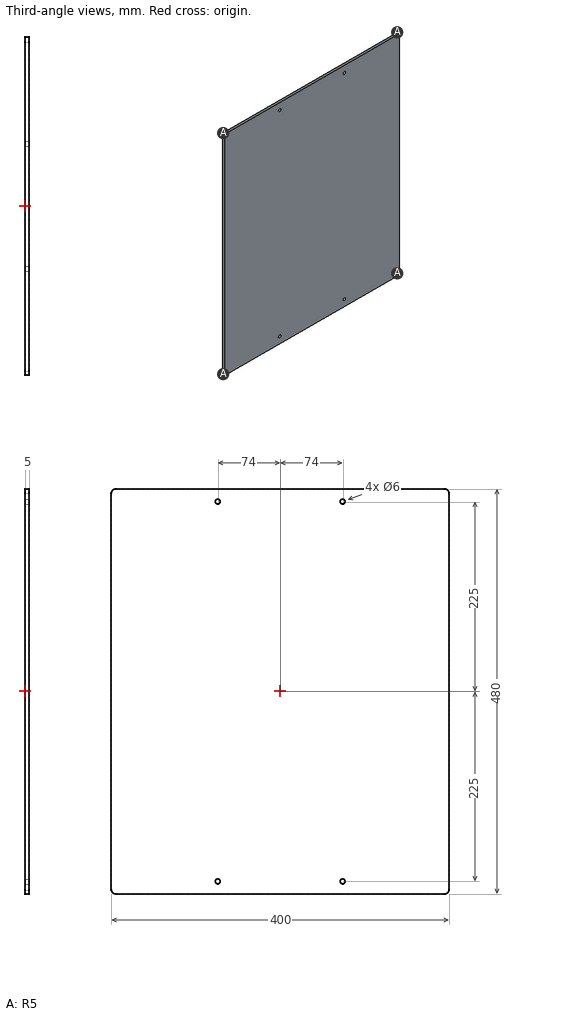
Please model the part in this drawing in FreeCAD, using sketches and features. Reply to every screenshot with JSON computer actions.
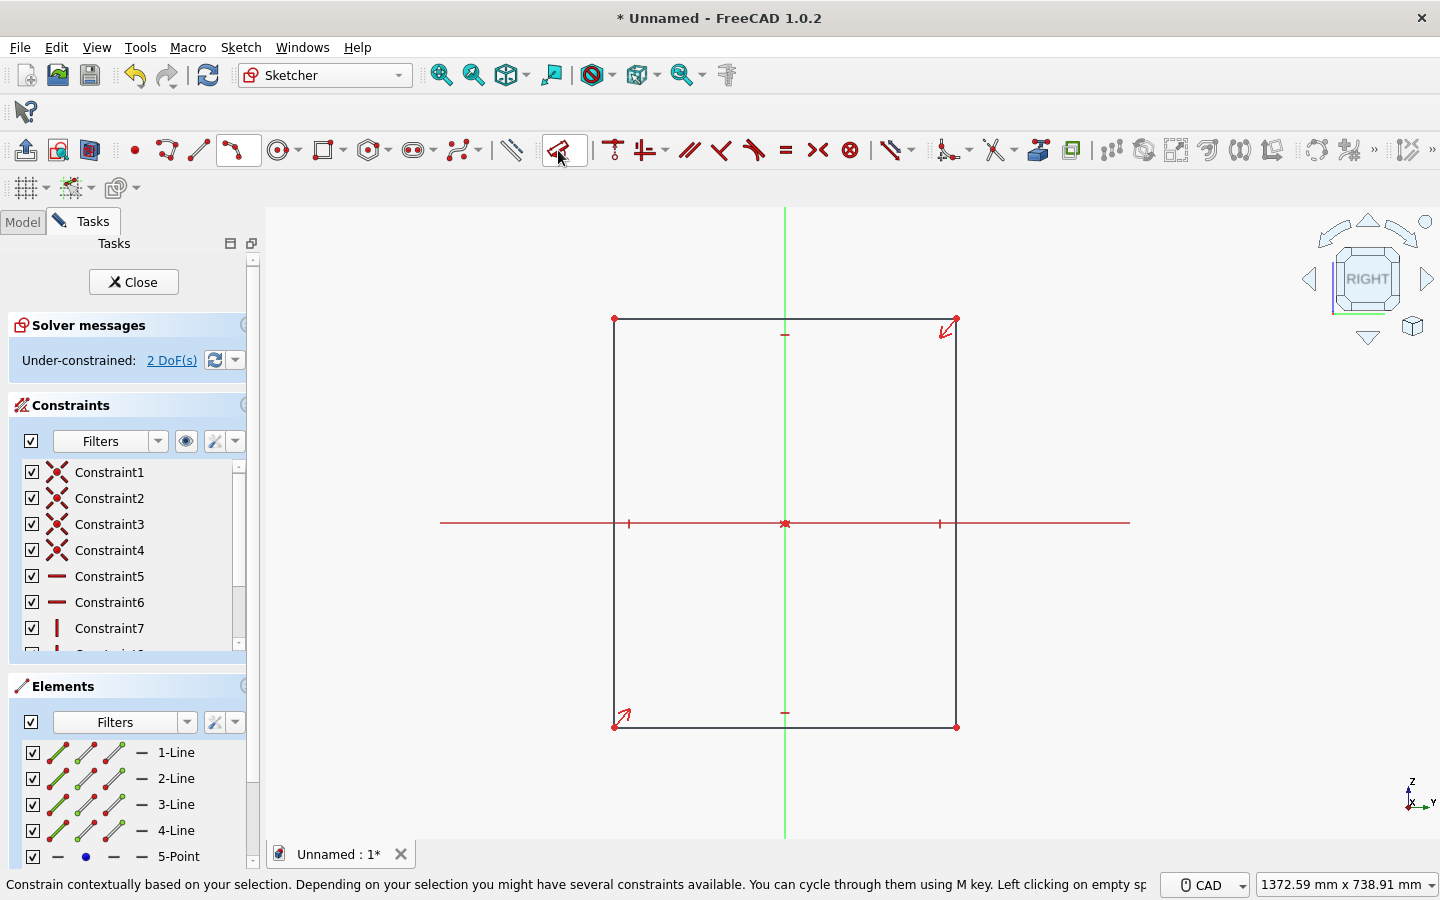
{"action": "left_click", "coordinate": [717, 728]}
{"action": "left_click", "coordinate": [706, 762]}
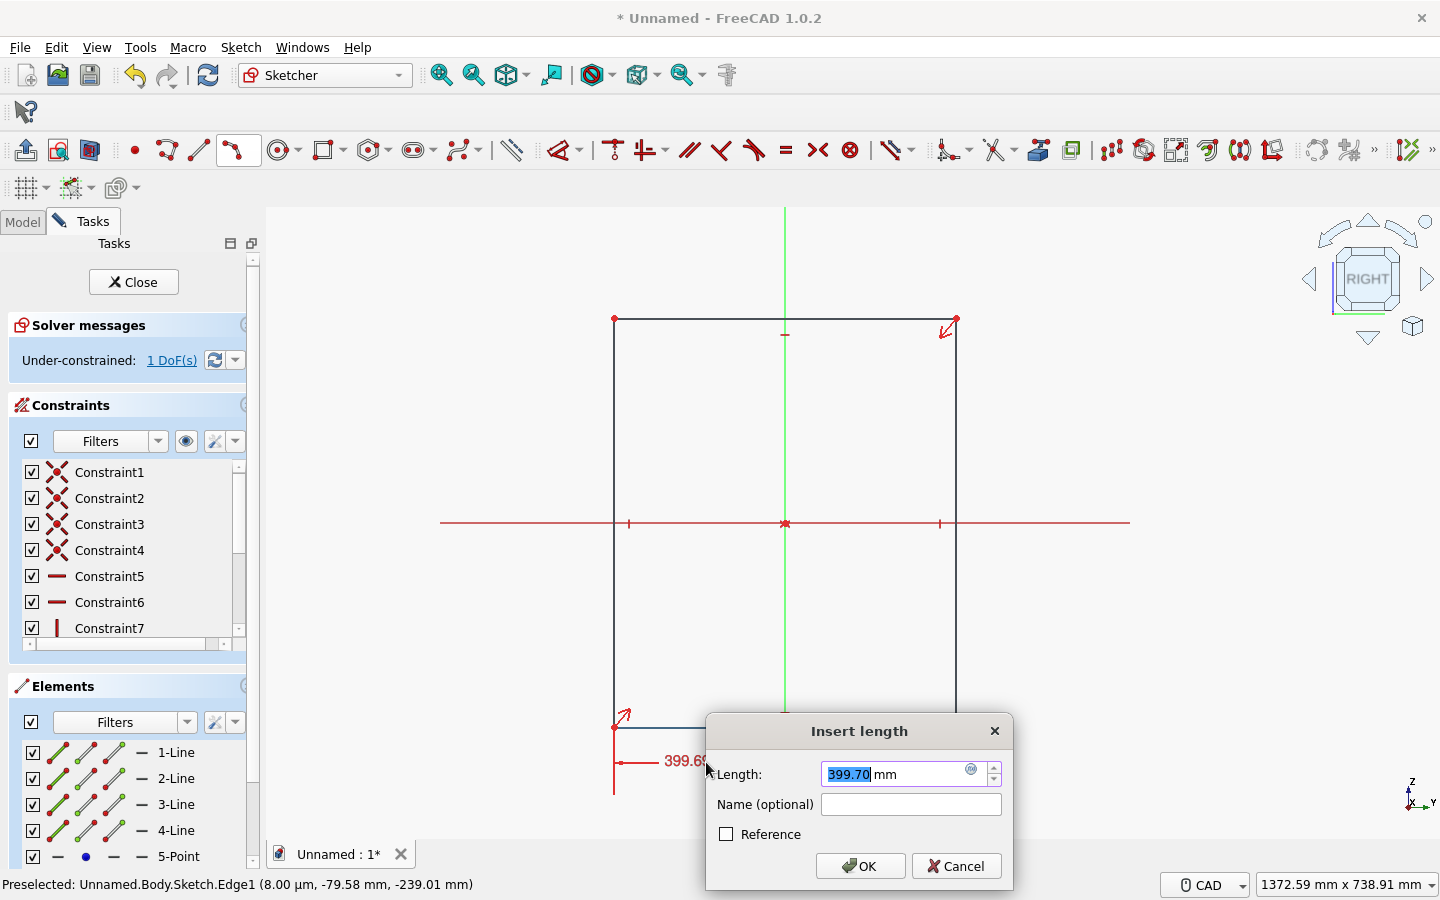
{"action": "type", "text": "400"}
{"action": "key", "text": "Return"}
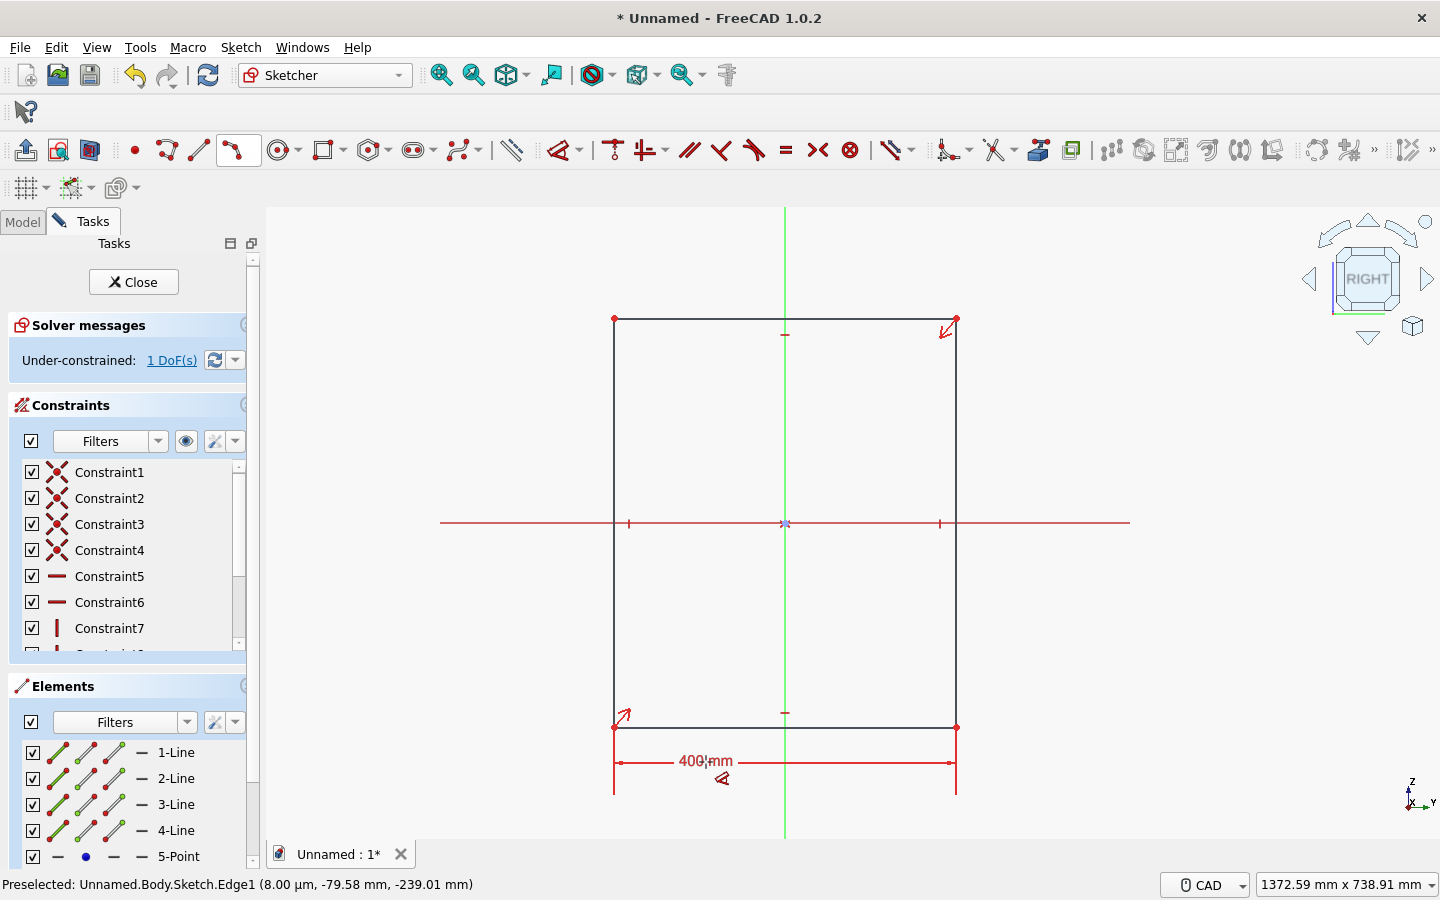
{"action": "left_click", "coordinate": [956, 605]}
{"action": "left_click", "coordinate": [990, 429]}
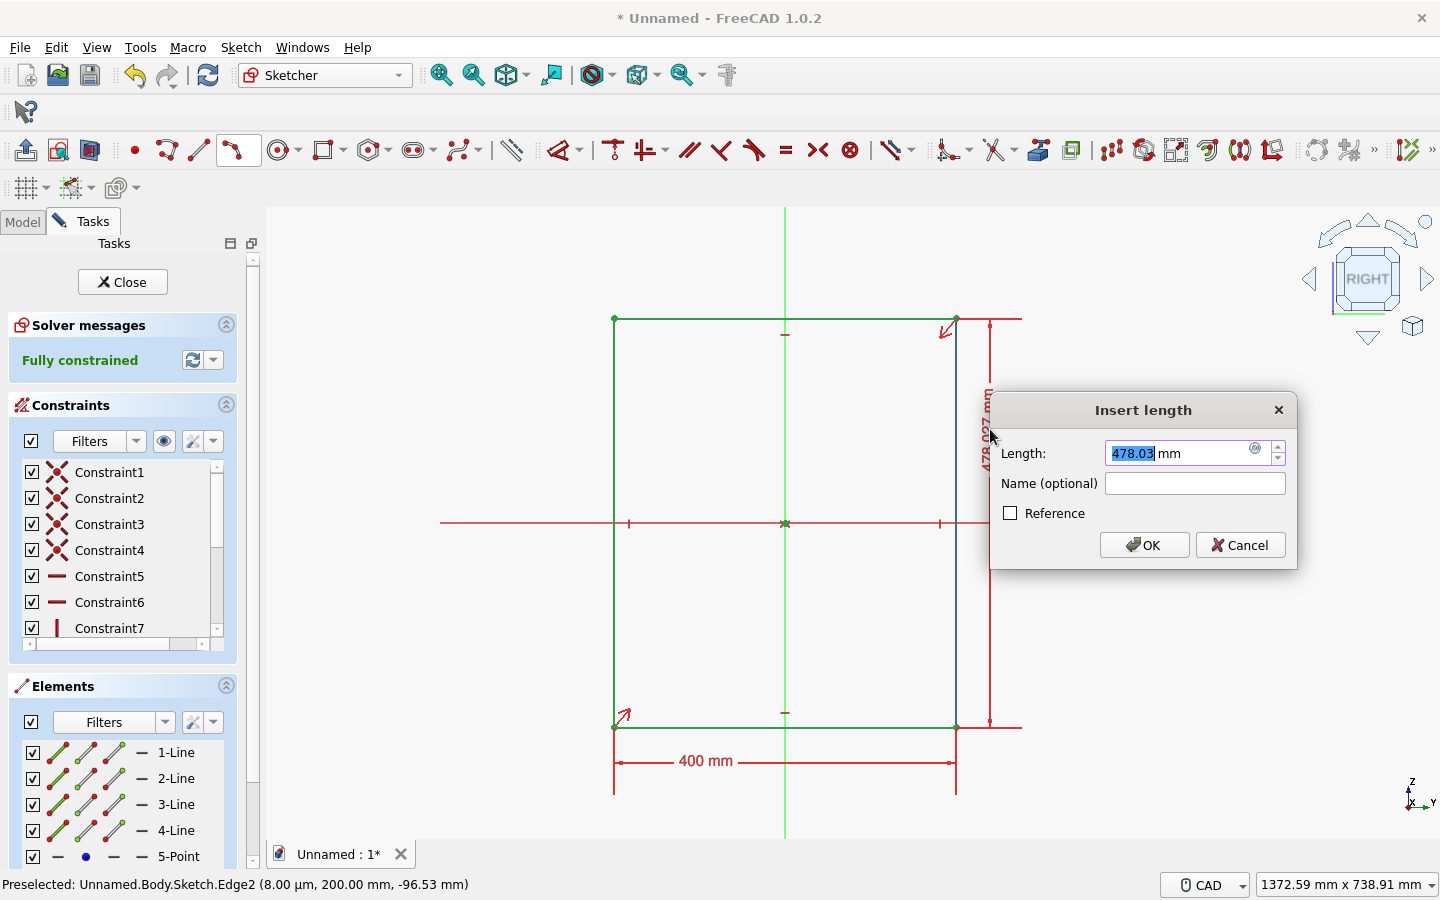
{"action": "type", "text": "480"}
{"action": "key", "text": "Return"}
{"action": "key", "text": "Escape"}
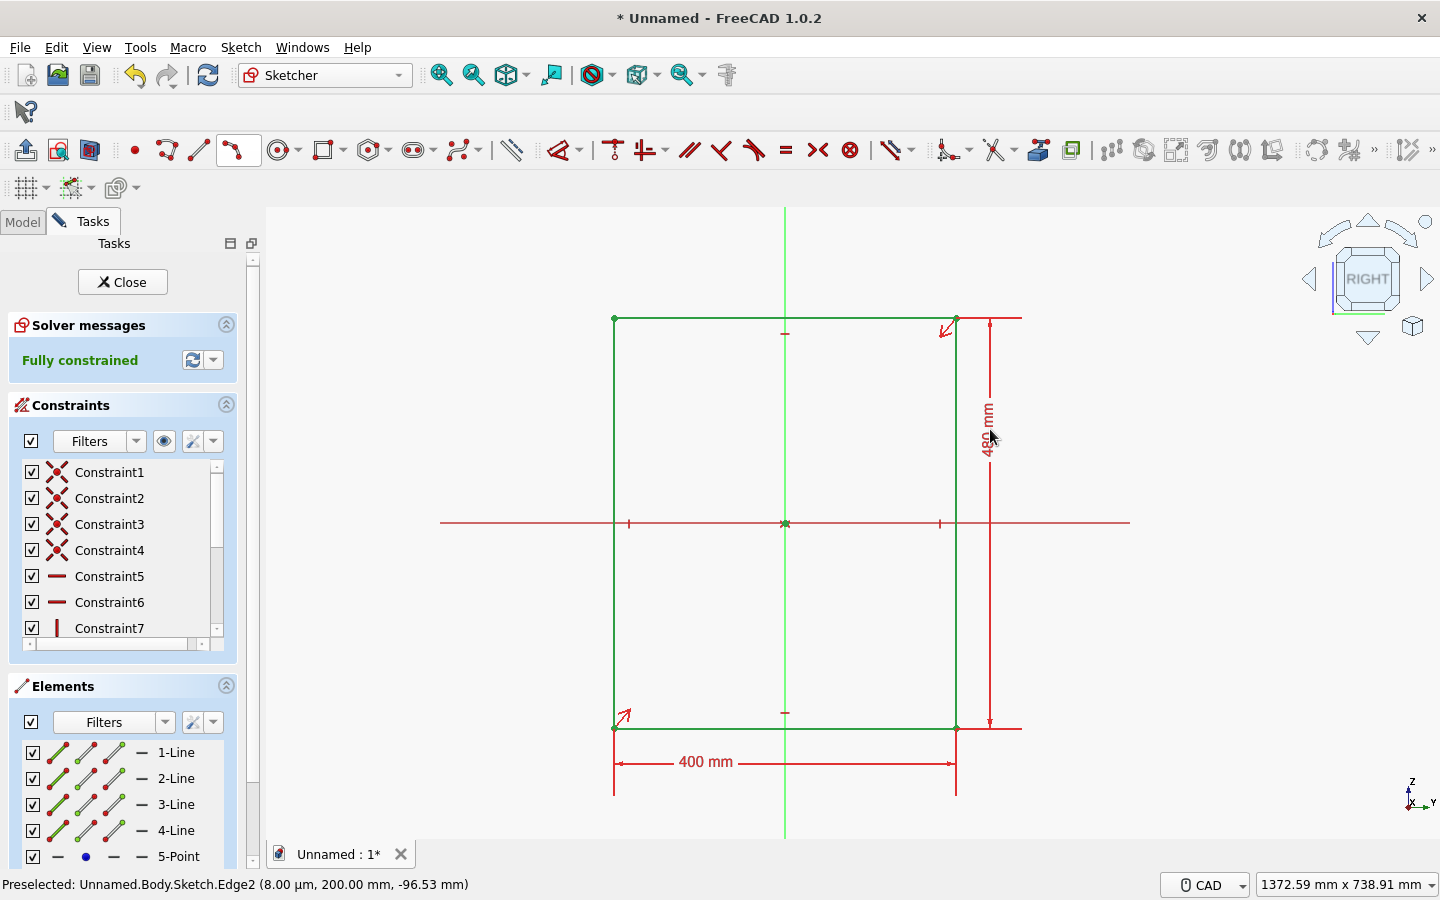
{"action": "left_click", "coordinate": [123, 282]}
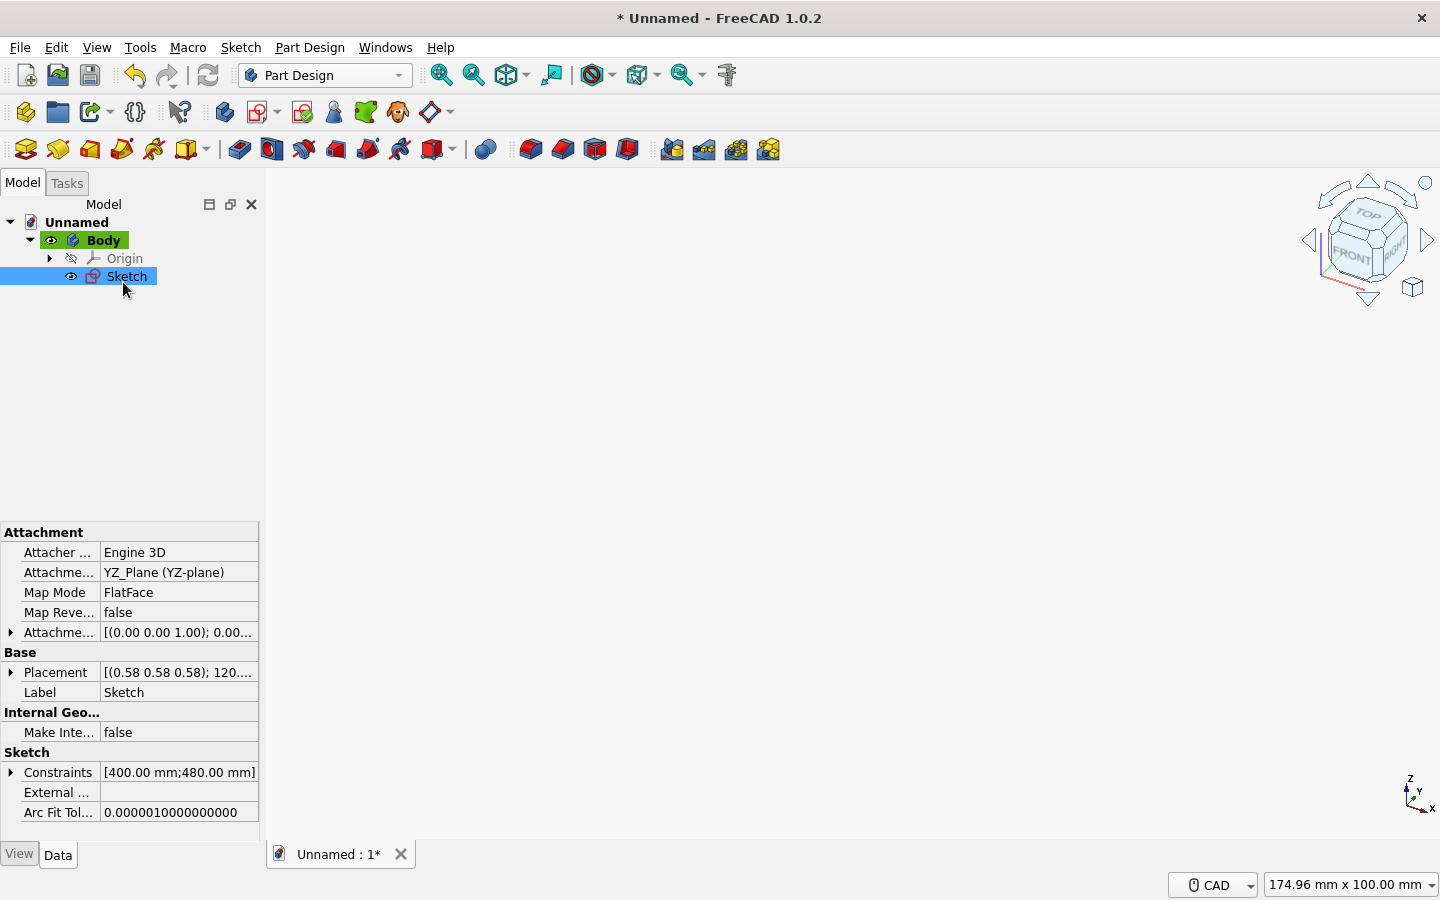
{"action": "left_click", "coordinate": [26, 150]}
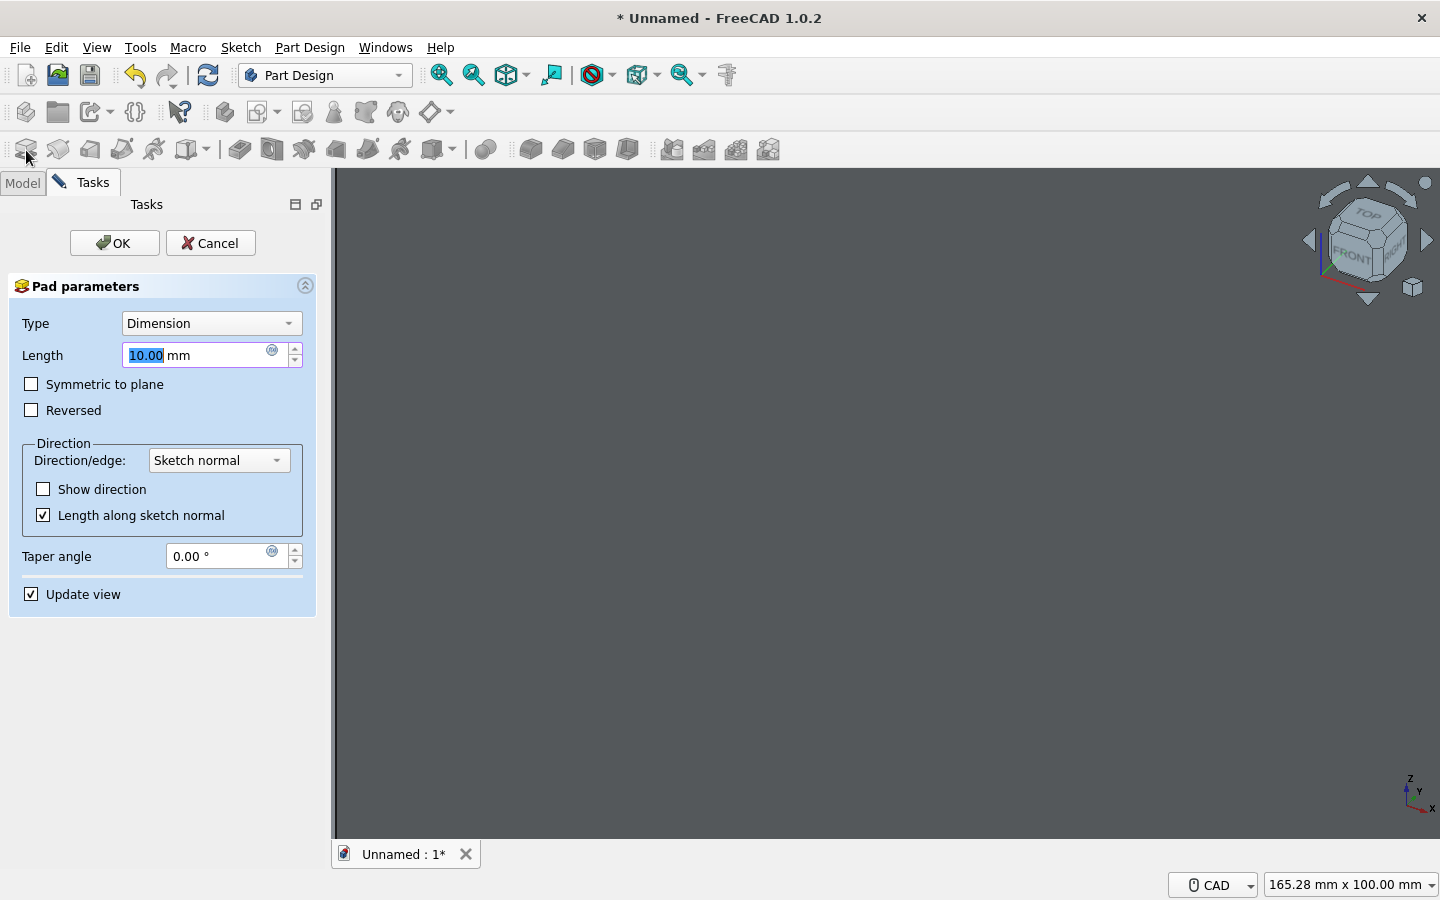
{"action": "type", "text": "5"}
{"action": "key", "text": "Tab"}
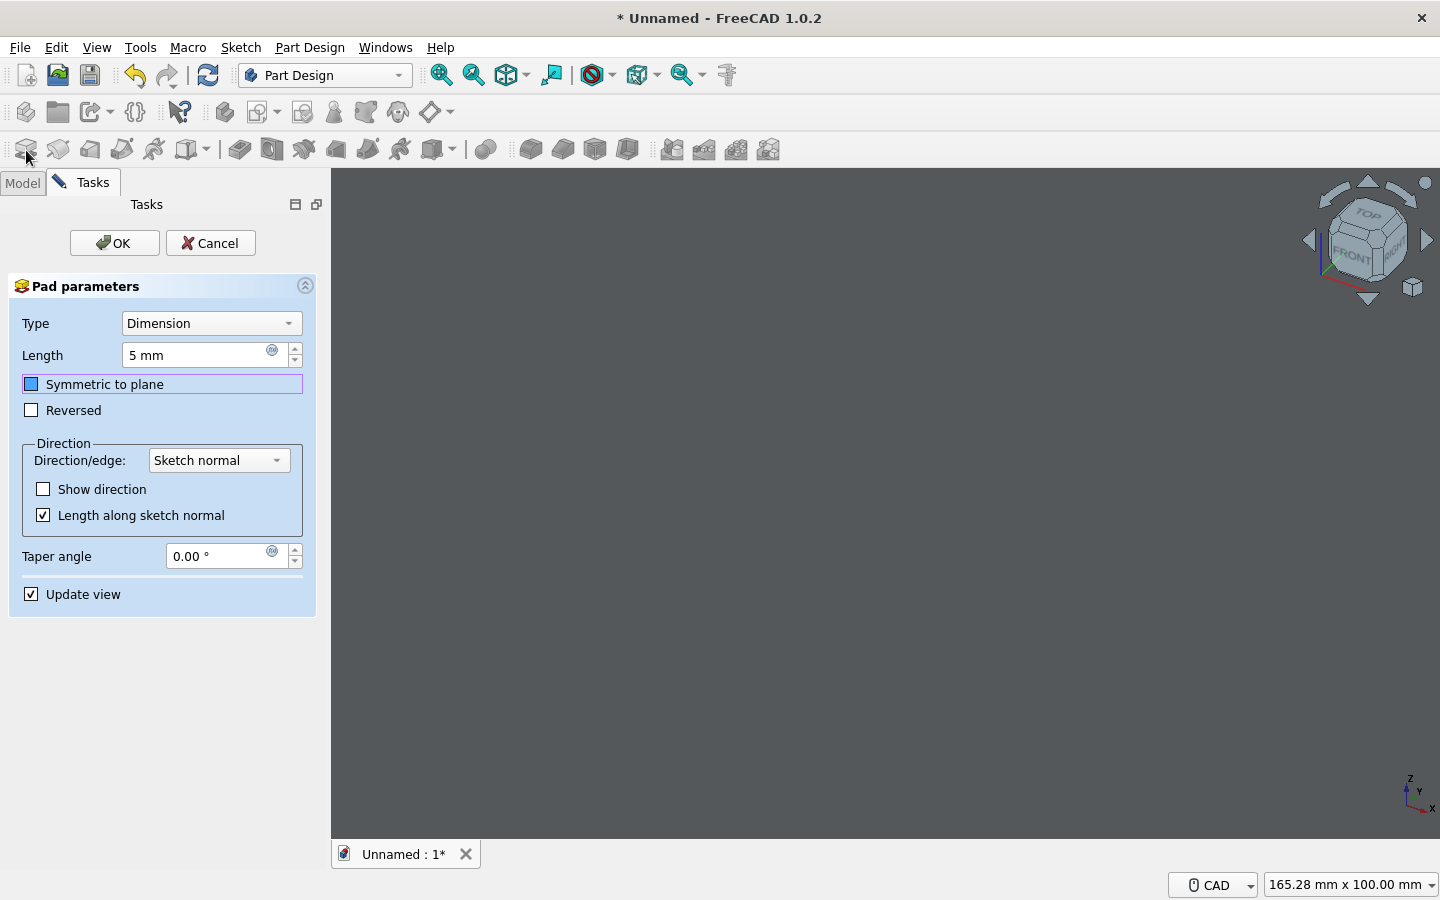
{"action": "left_click", "coordinate": [115, 243]}